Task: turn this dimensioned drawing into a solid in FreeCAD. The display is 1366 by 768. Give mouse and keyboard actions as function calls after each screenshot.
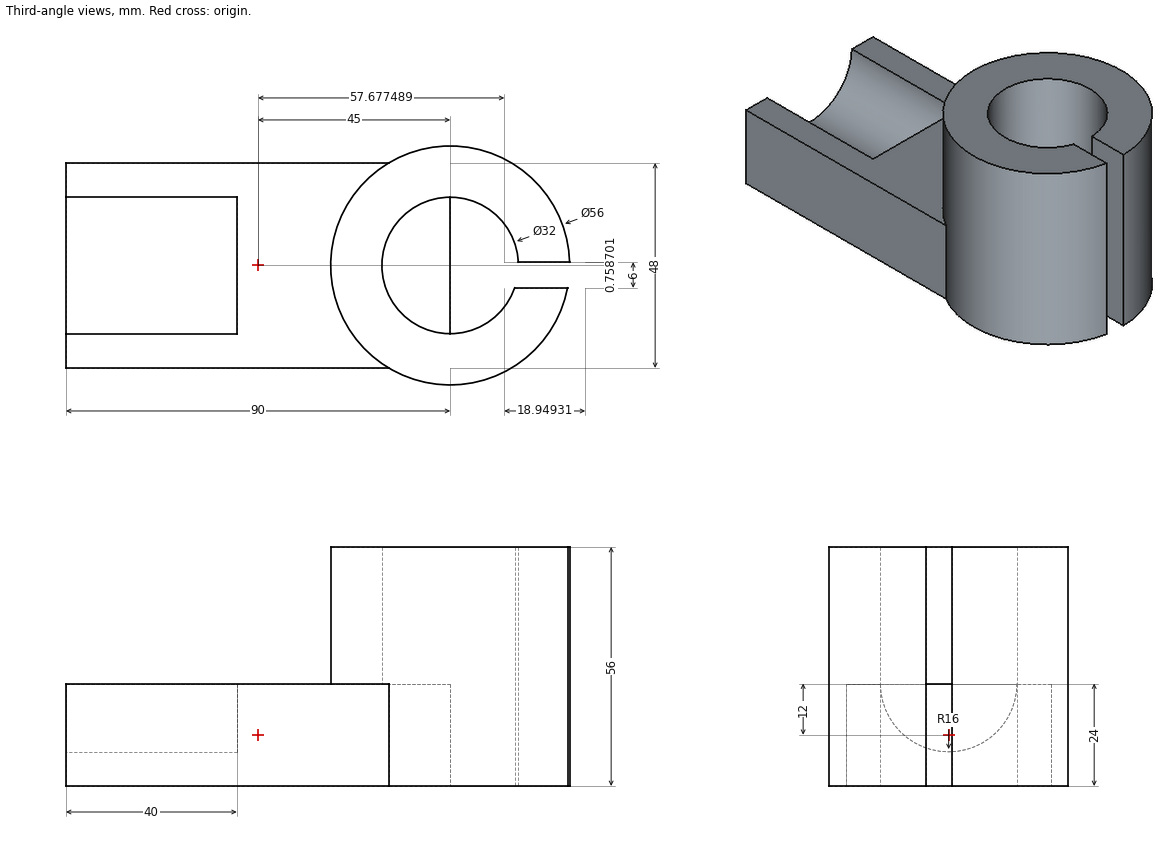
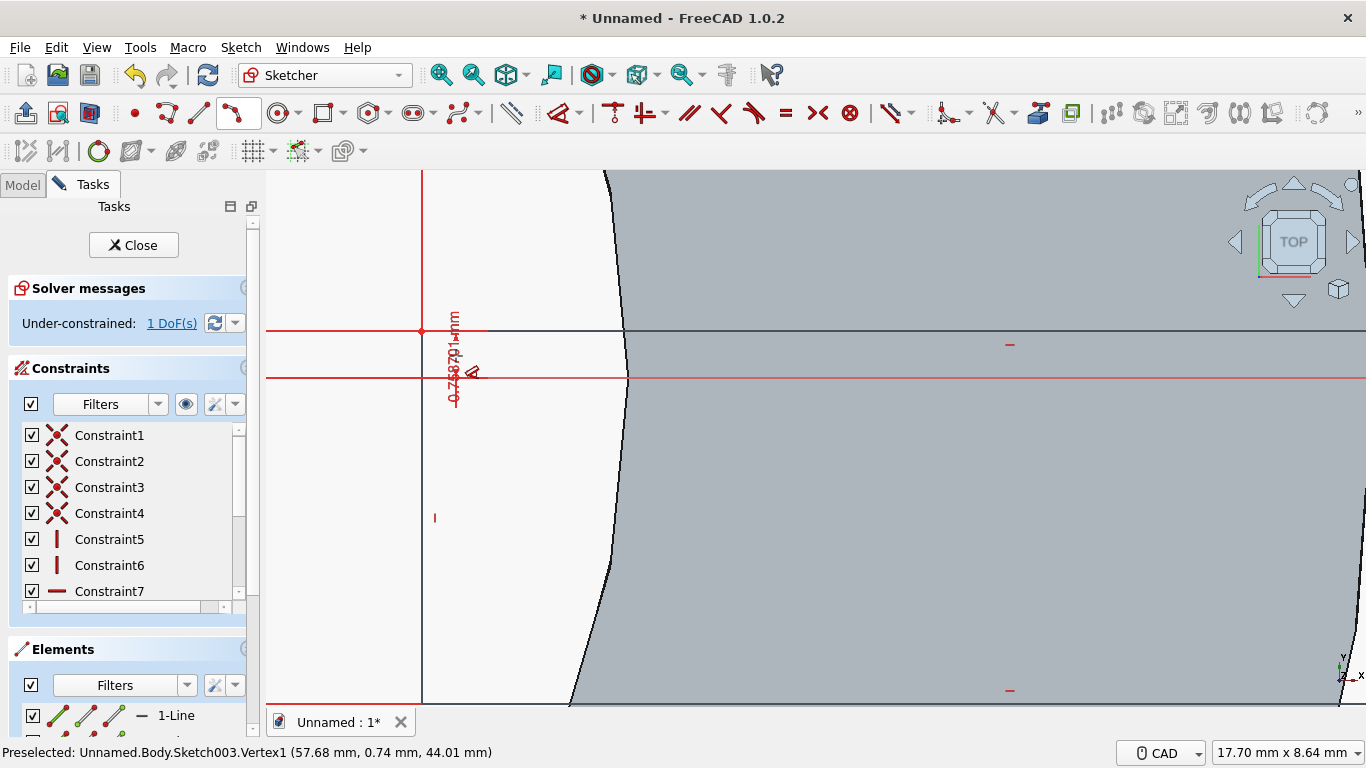
click(422, 331)
click(358, 297)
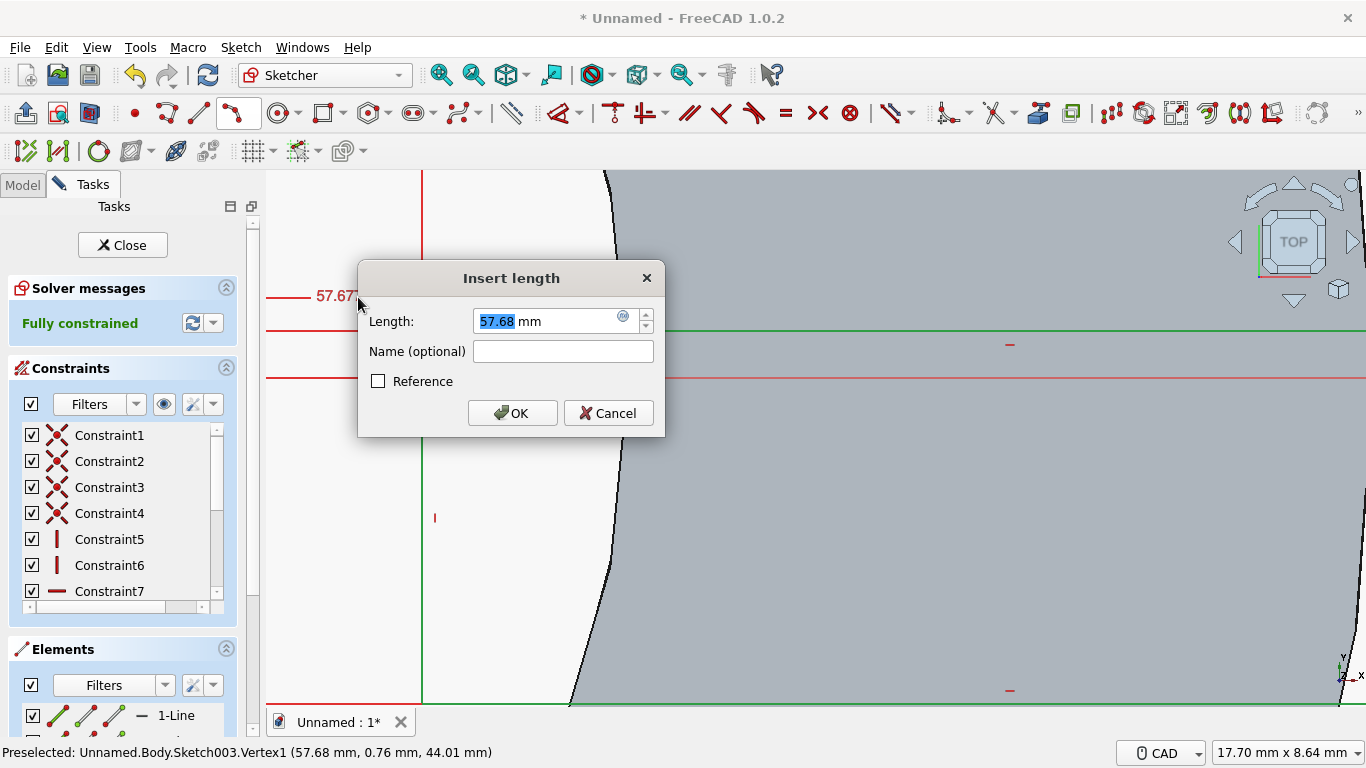
text(57.677489)
key(Return)
key(Escape)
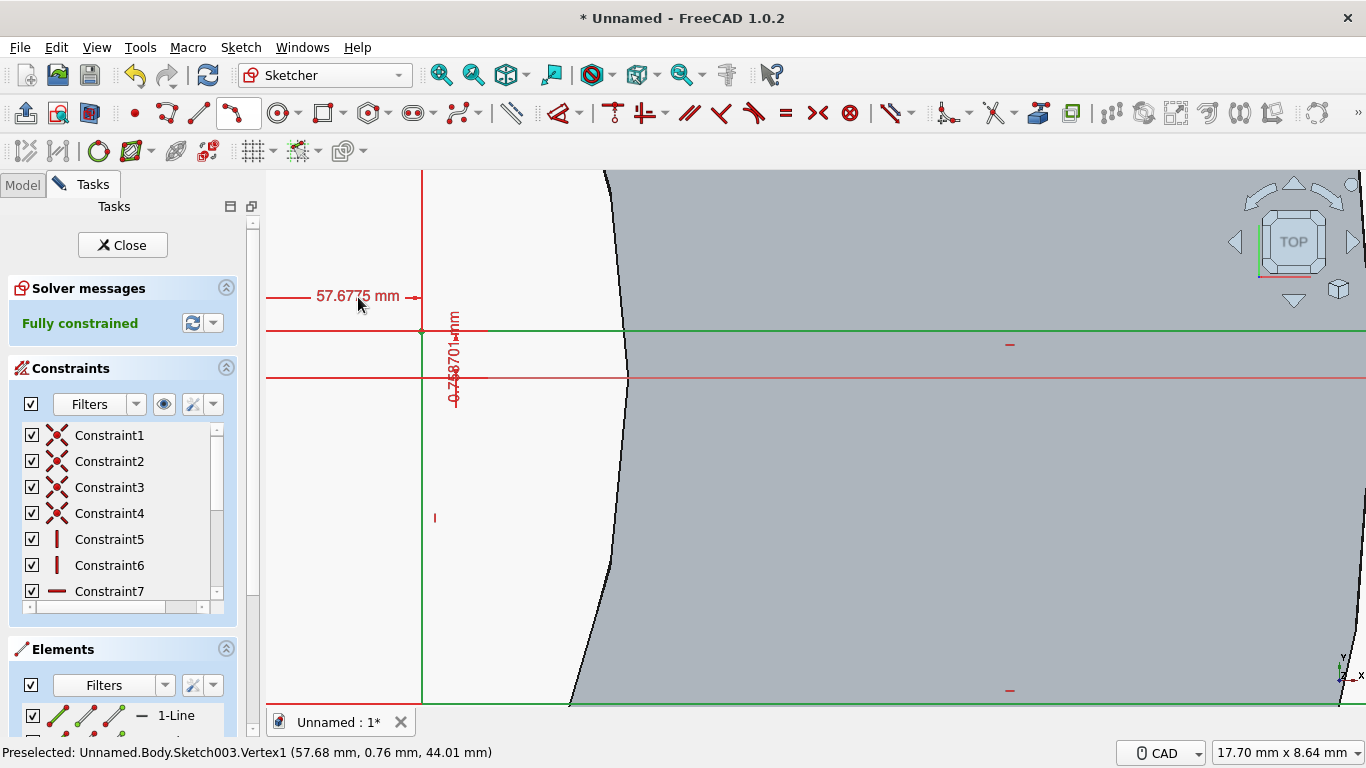
click(123, 245)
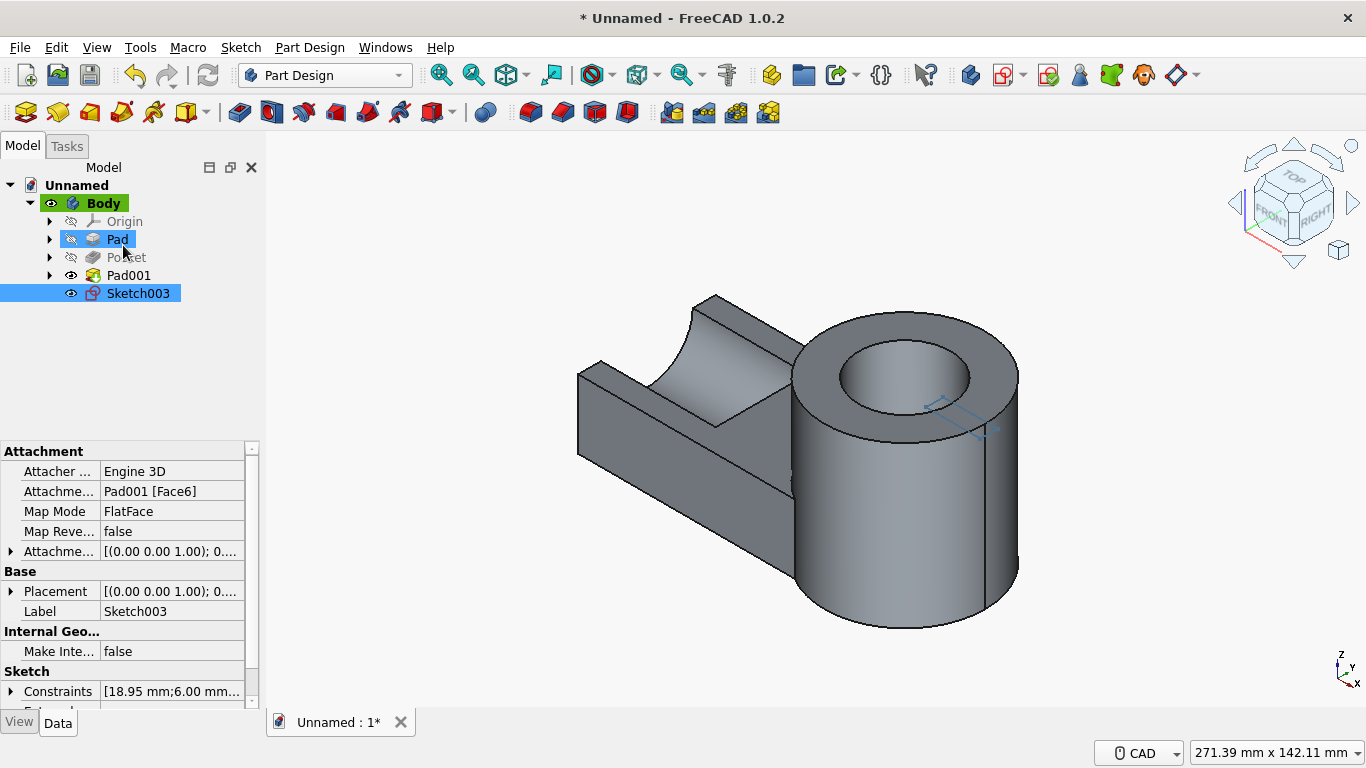
click(240, 112)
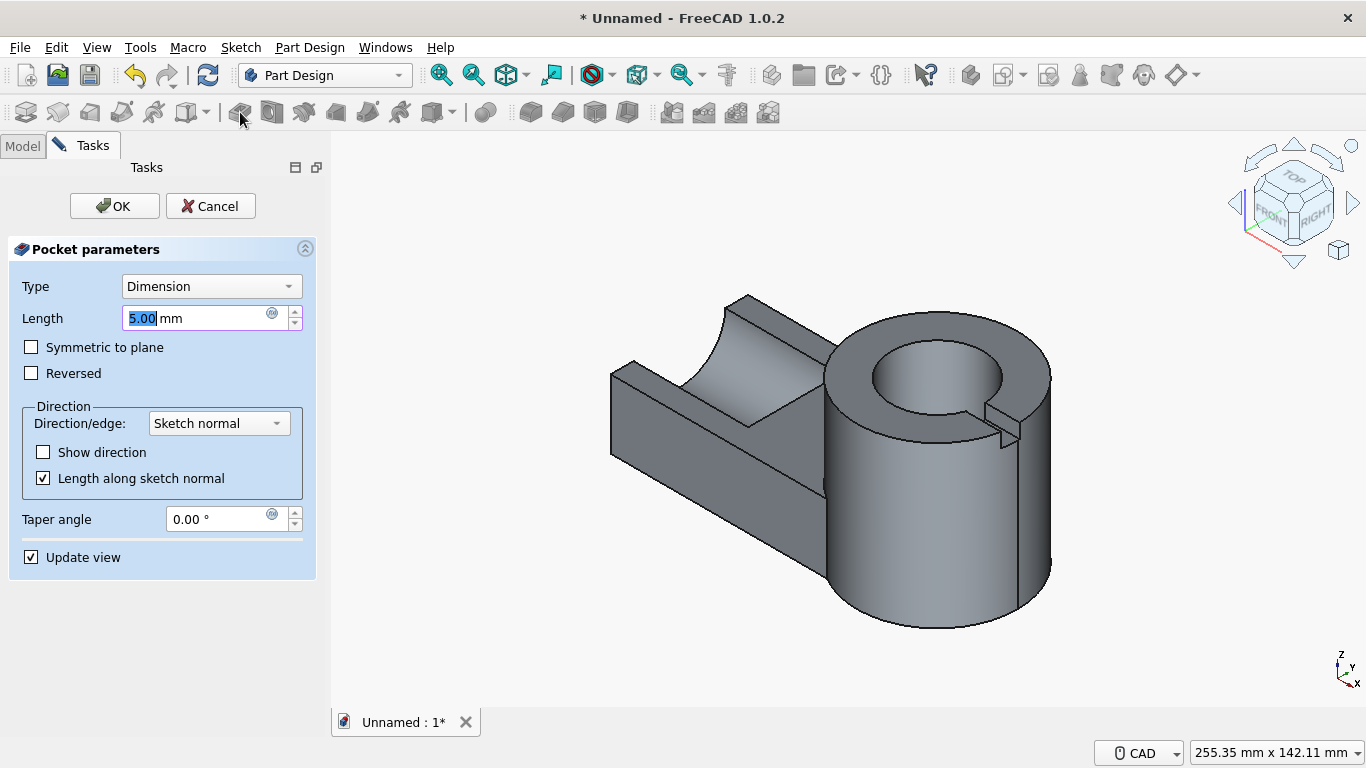
text(56)
key(Tab)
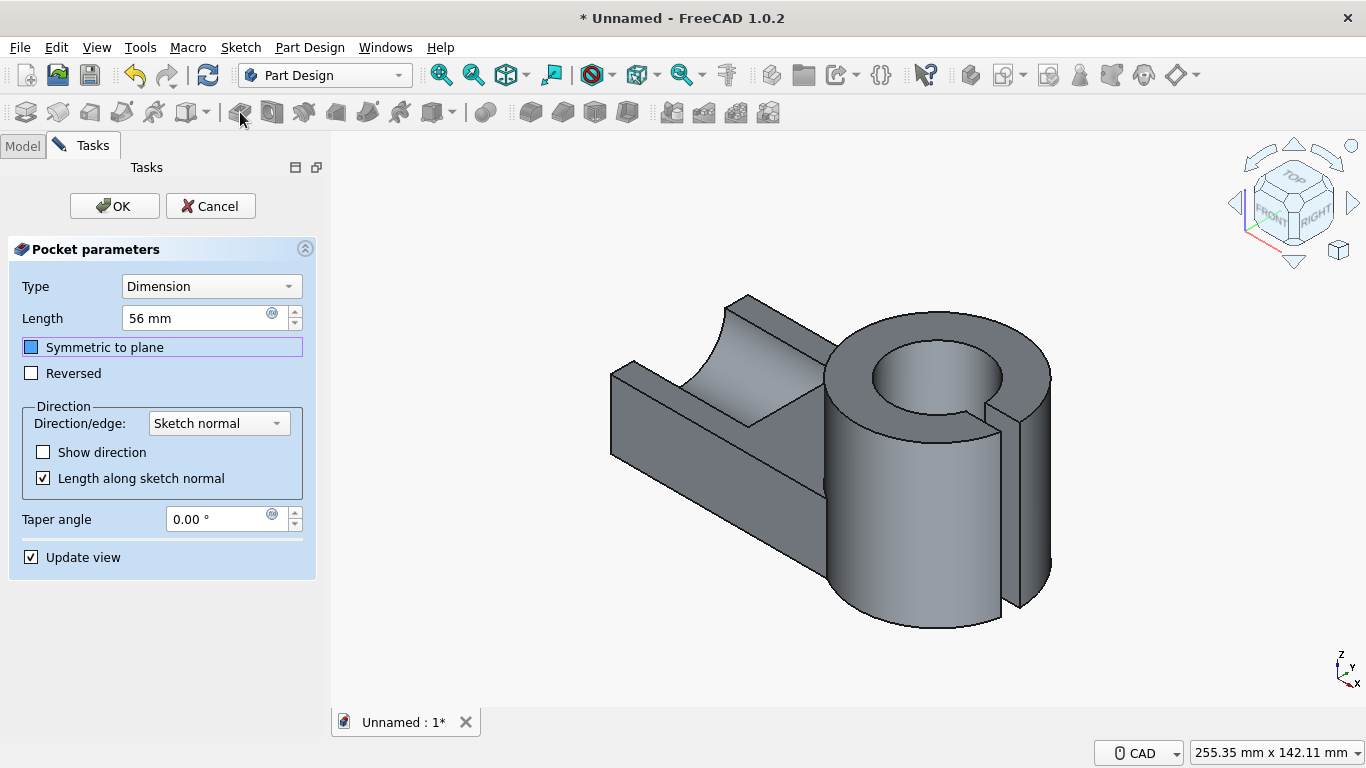
click(115, 206)